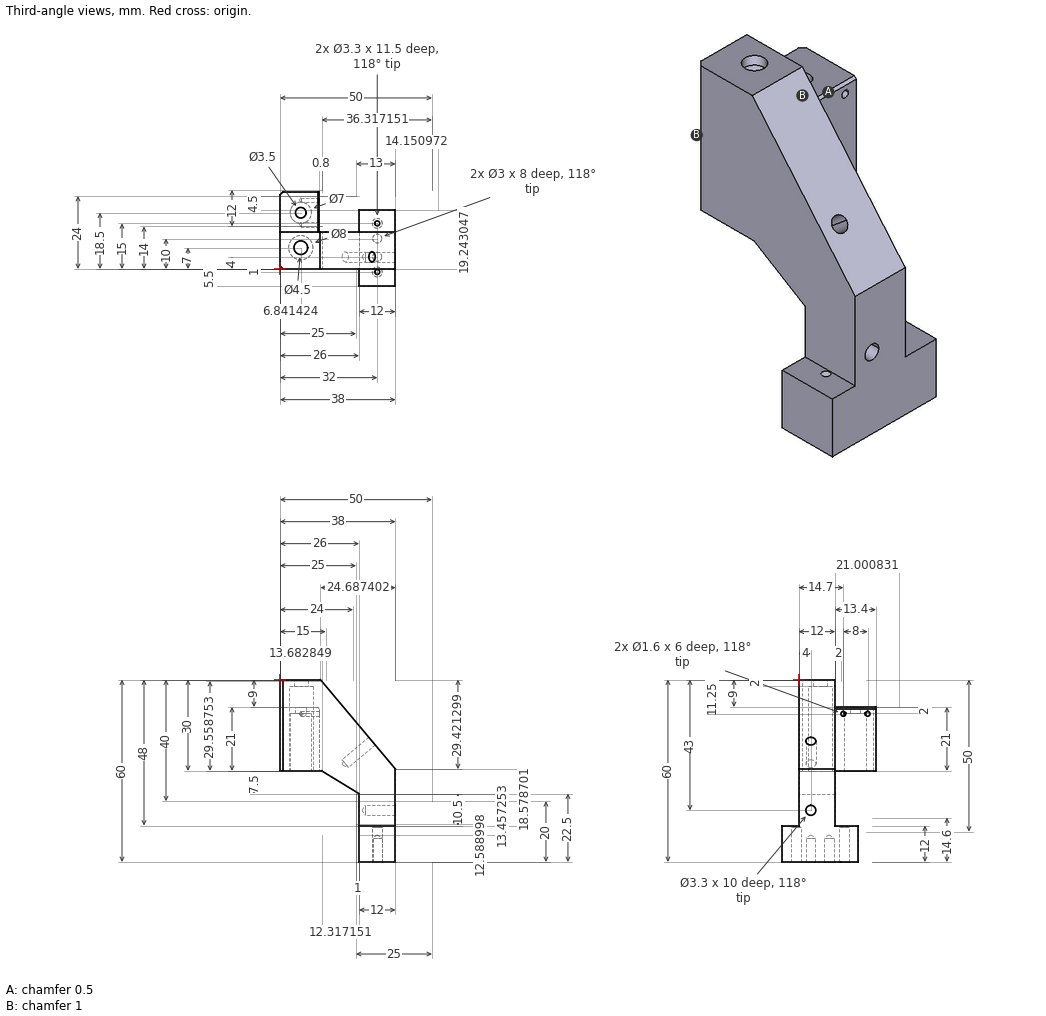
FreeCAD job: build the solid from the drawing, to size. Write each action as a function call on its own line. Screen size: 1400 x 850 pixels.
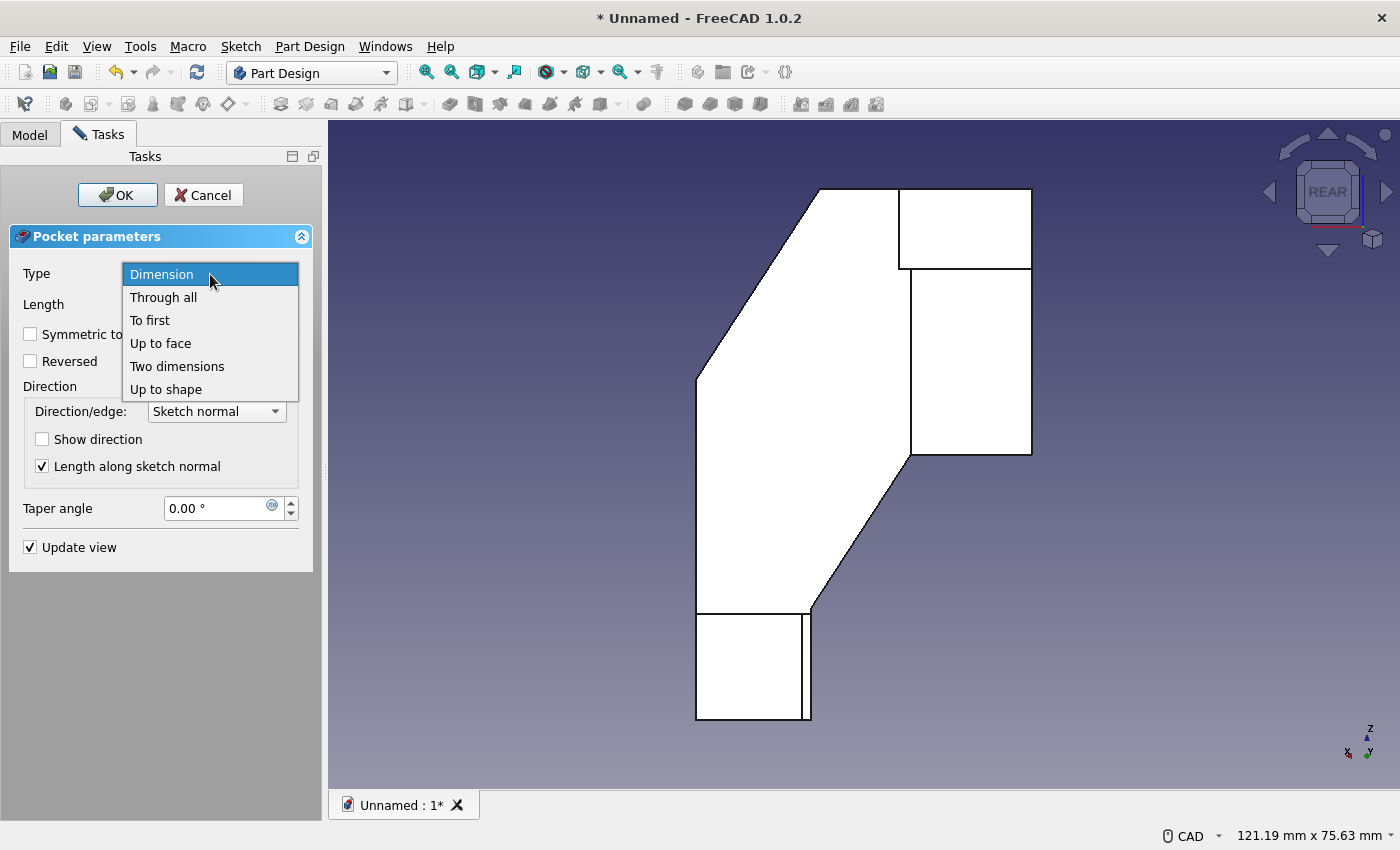
click(208, 298)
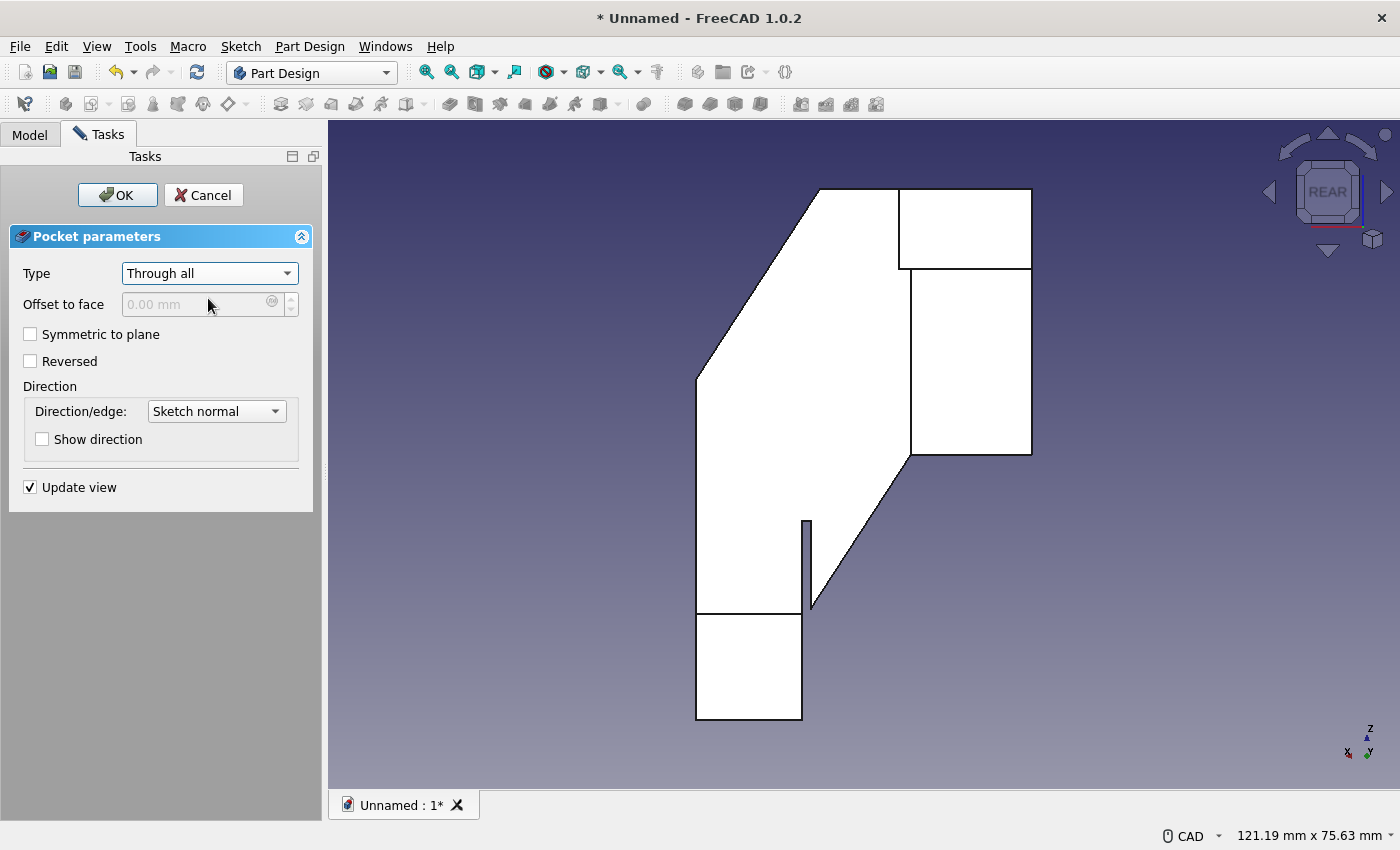
click(118, 195)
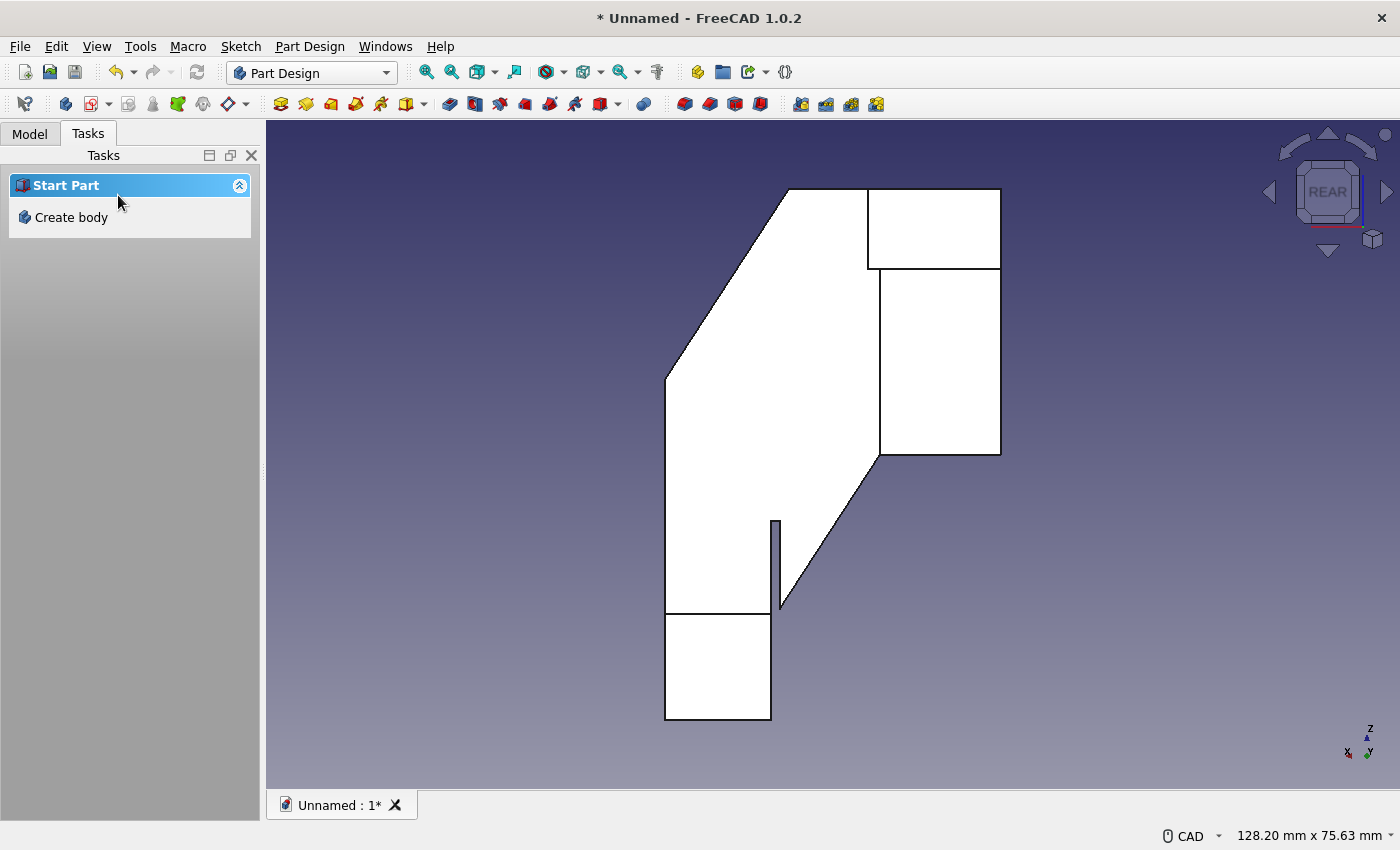
click(772, 400)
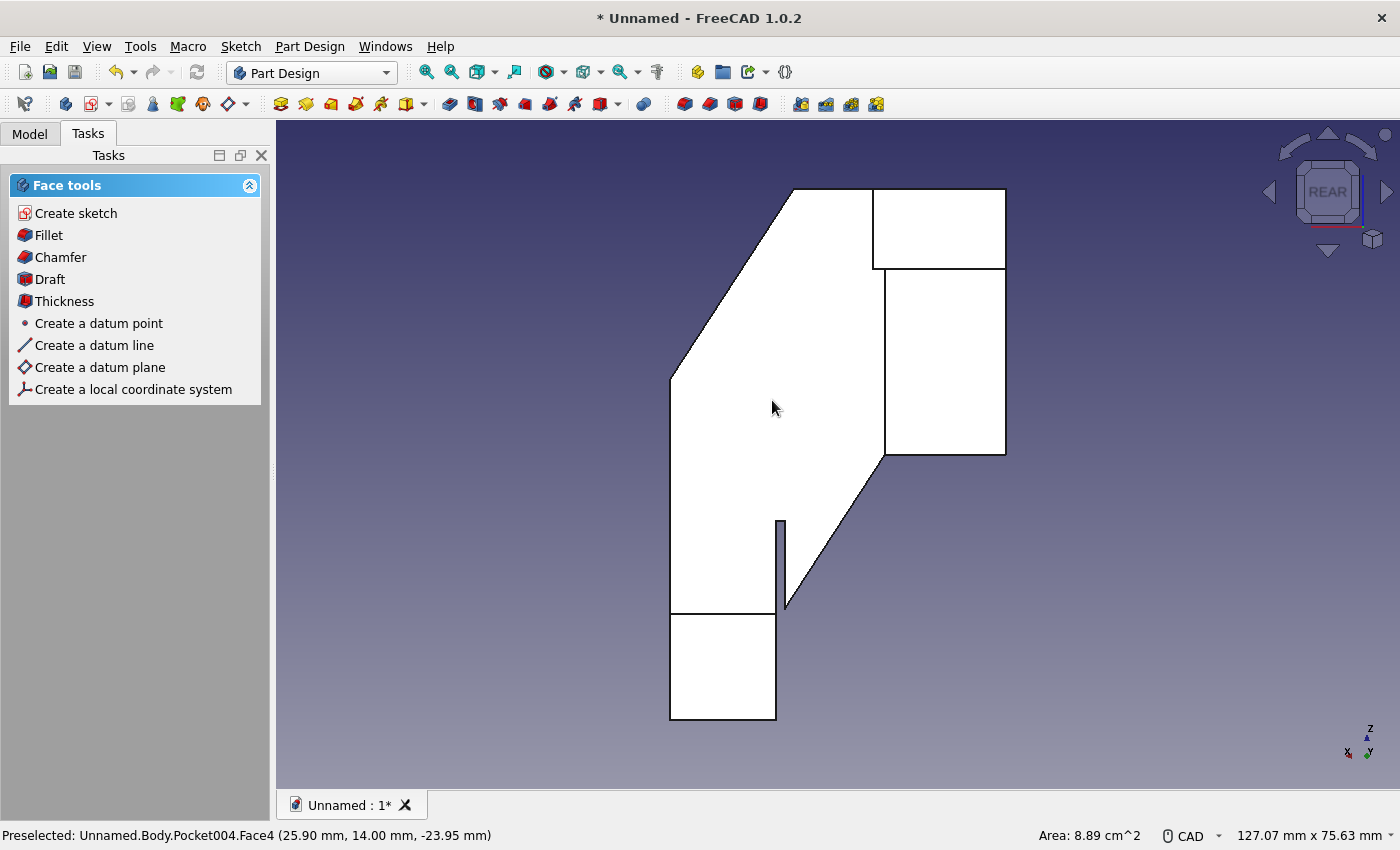
click(90, 104)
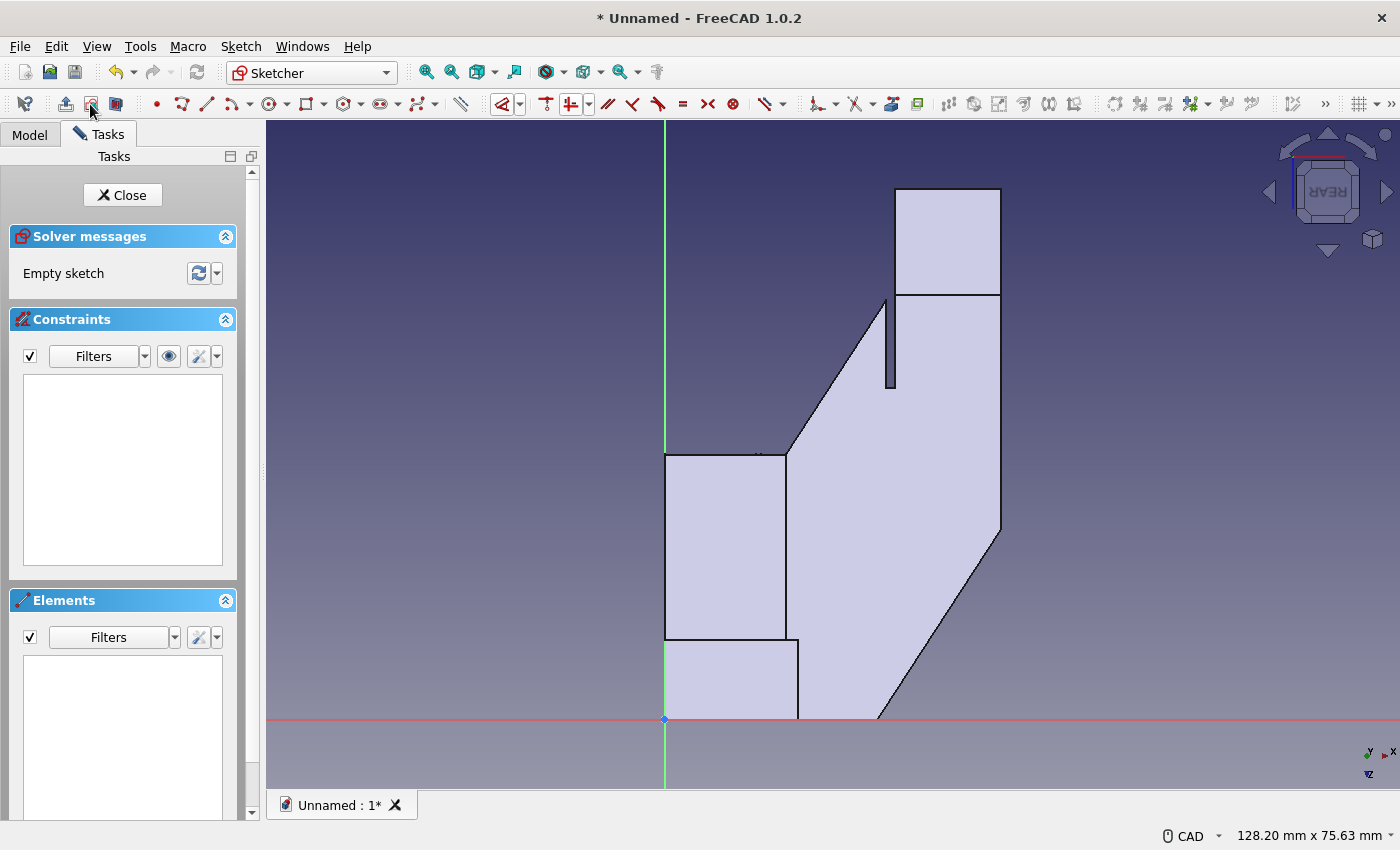
click(182, 104)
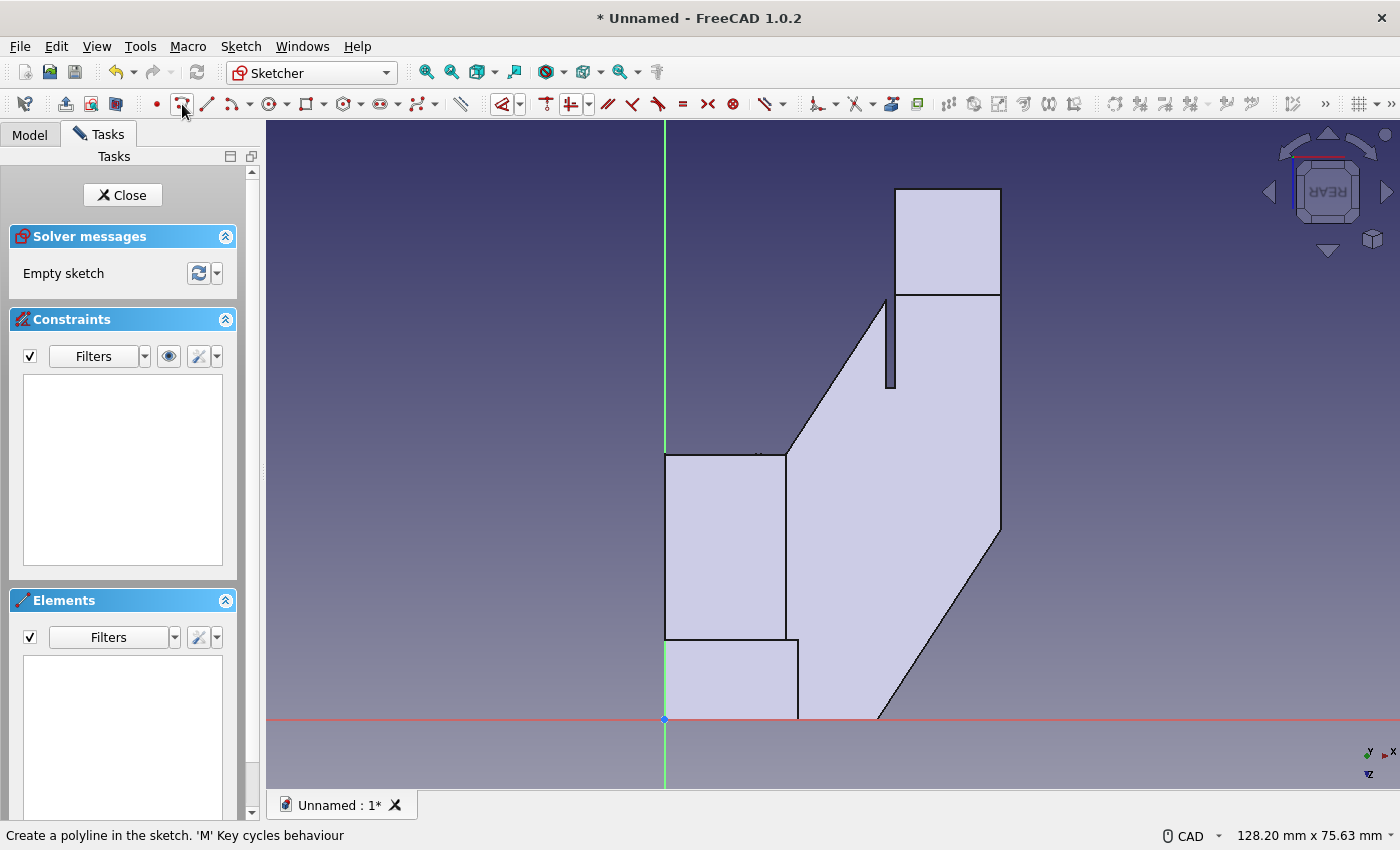
click(786, 454)
click(895, 388)
click(895, 269)
click(786, 269)
click(786, 455)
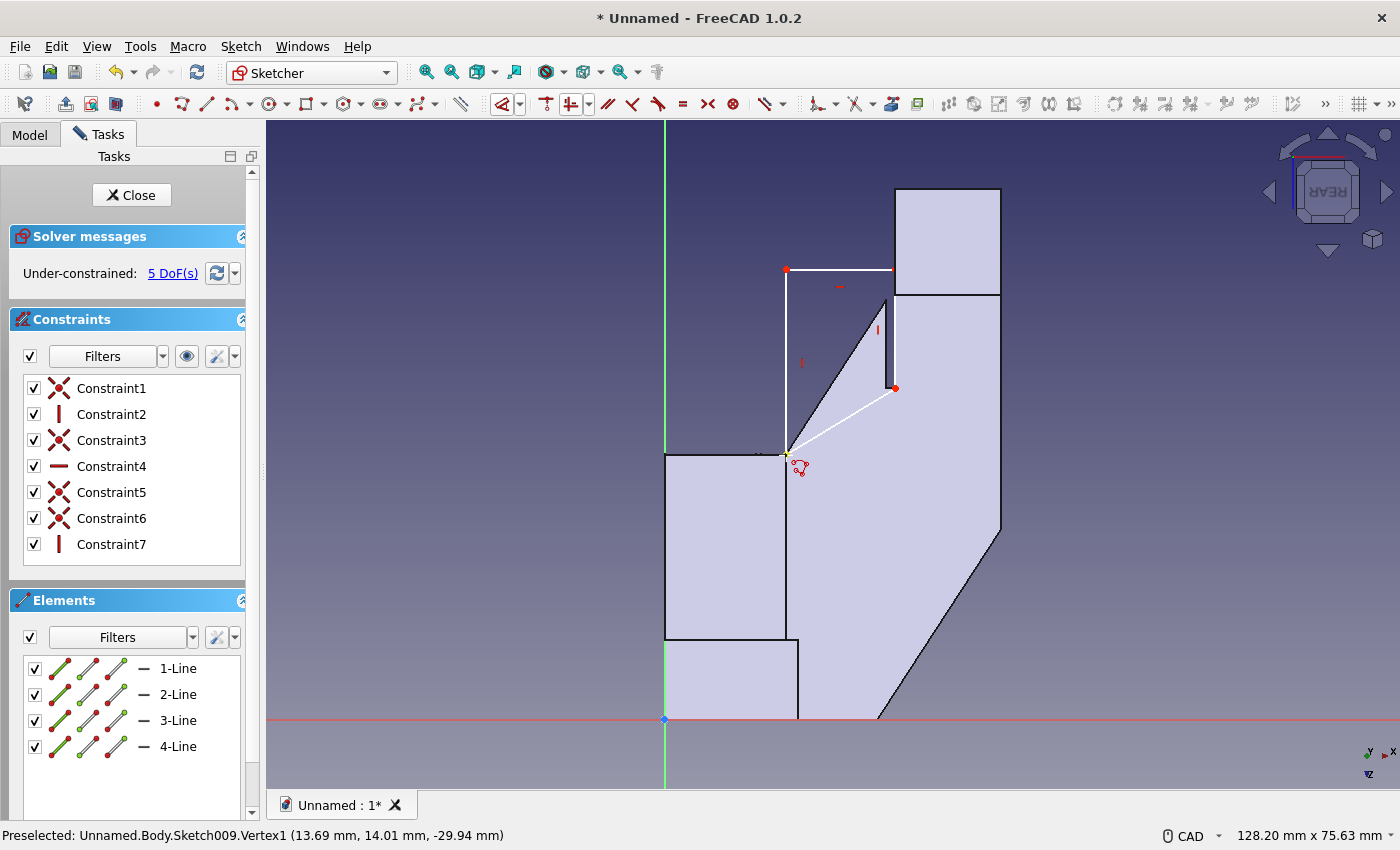
click(783, 720)
click(1001, 711)
click(1001, 460)
click(783, 720)
key(Escape)
key(Escape)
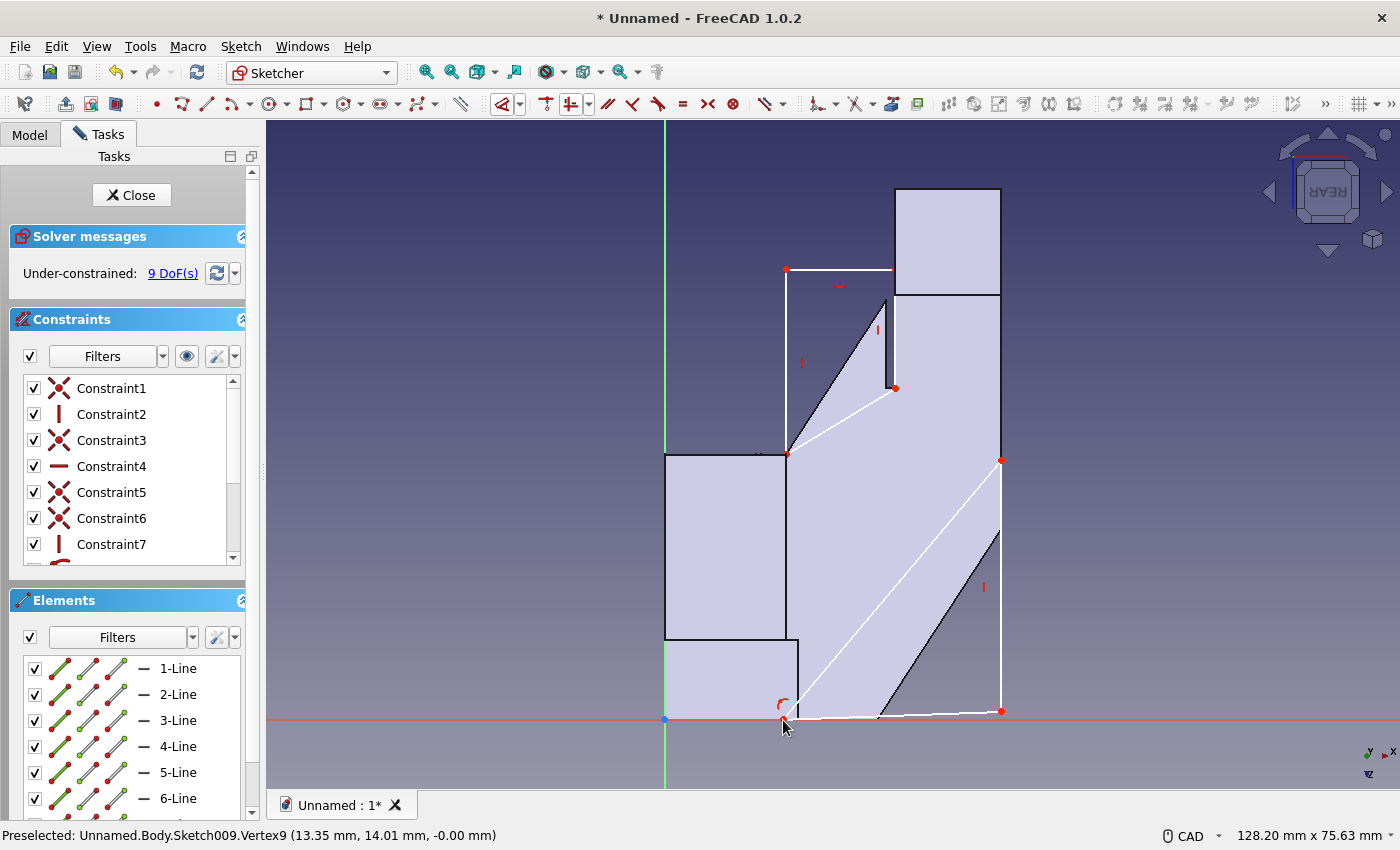
click(848, 718)